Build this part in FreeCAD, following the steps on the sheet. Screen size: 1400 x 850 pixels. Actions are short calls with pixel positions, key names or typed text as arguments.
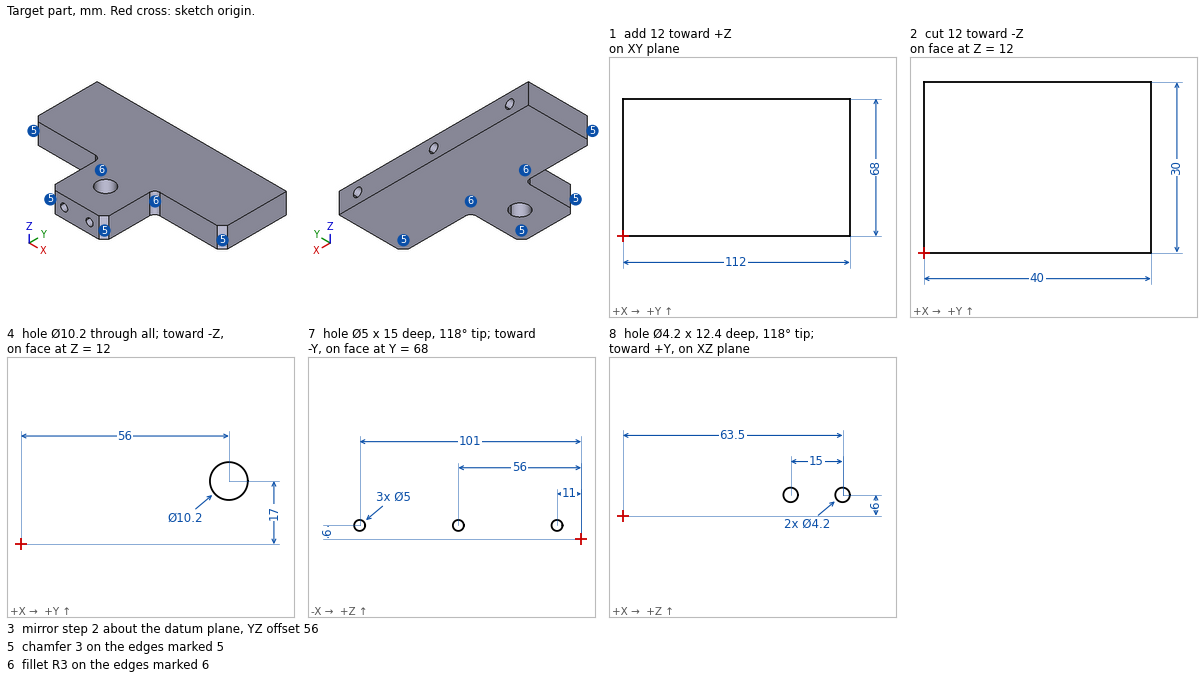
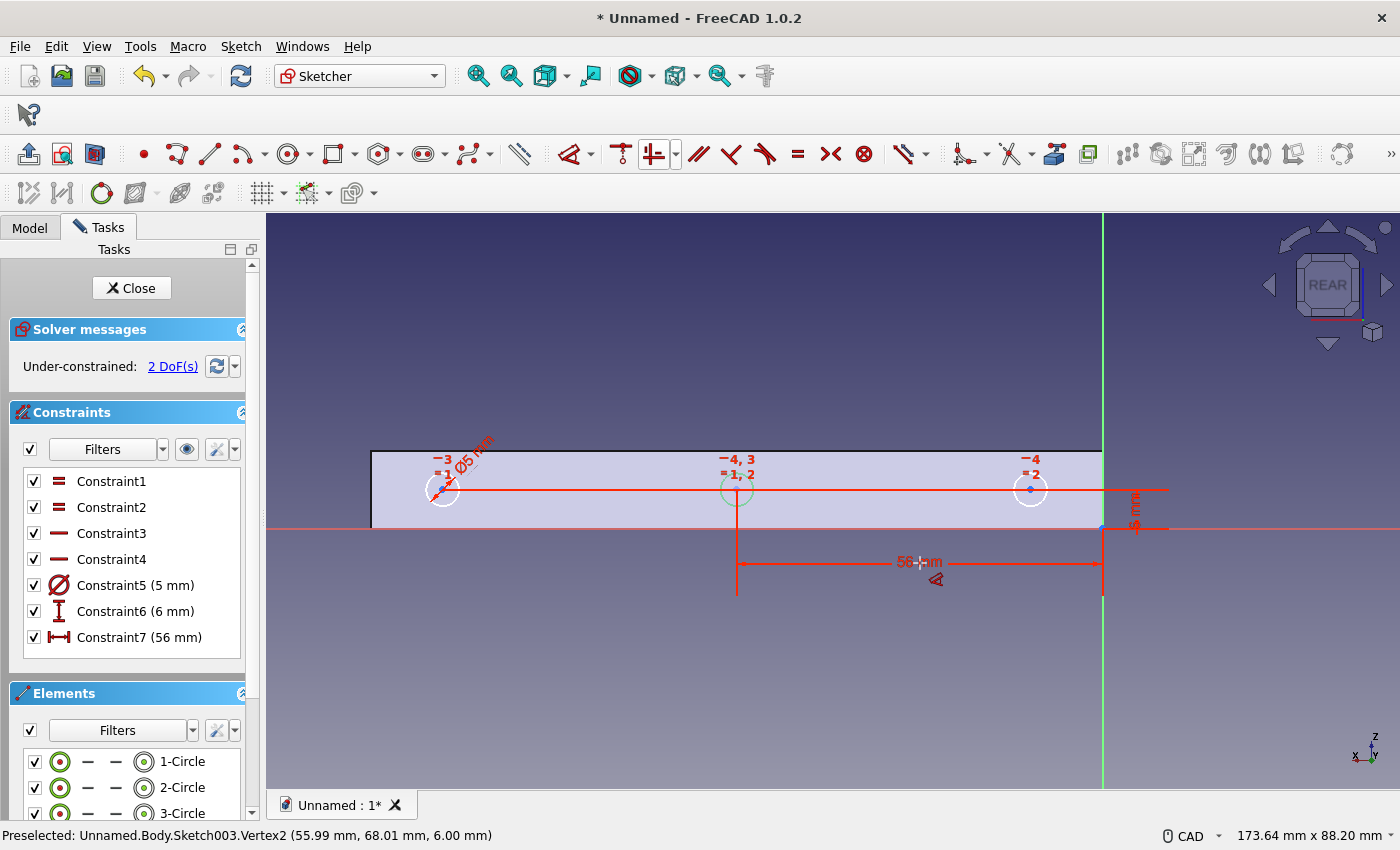
click(1031, 490)
click(1067, 563)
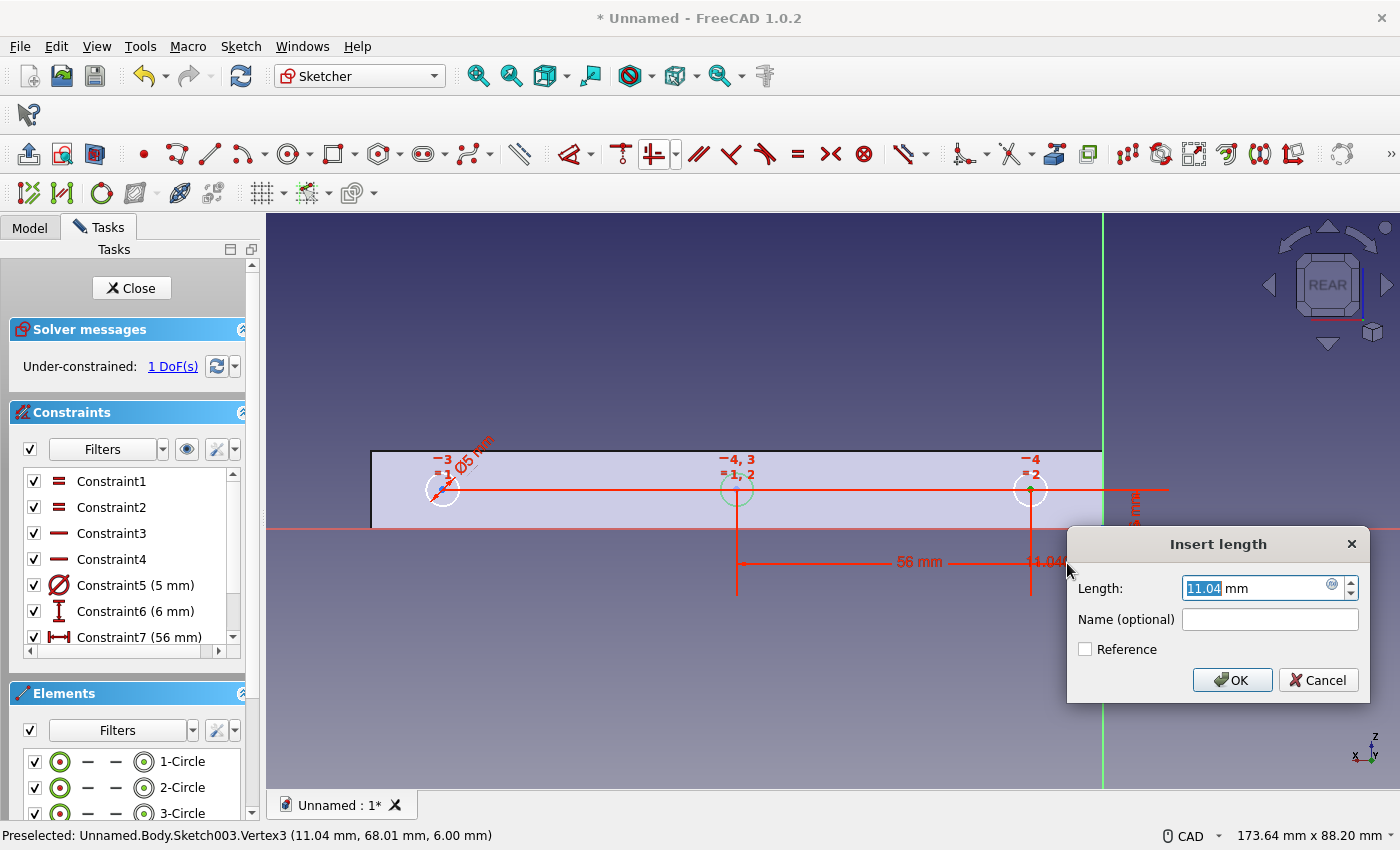
text(11)
key(Return)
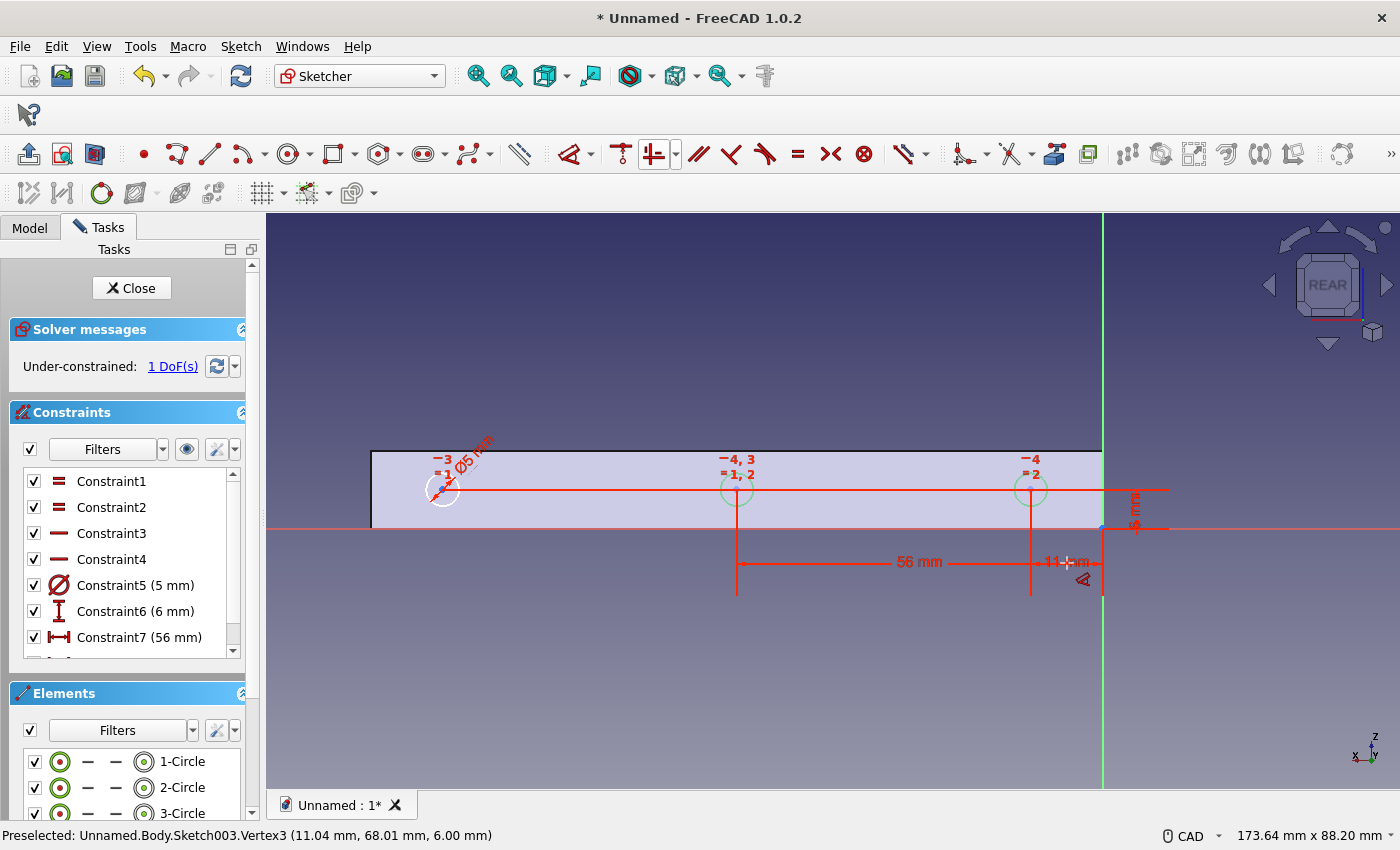
click(443, 490)
click(773, 563)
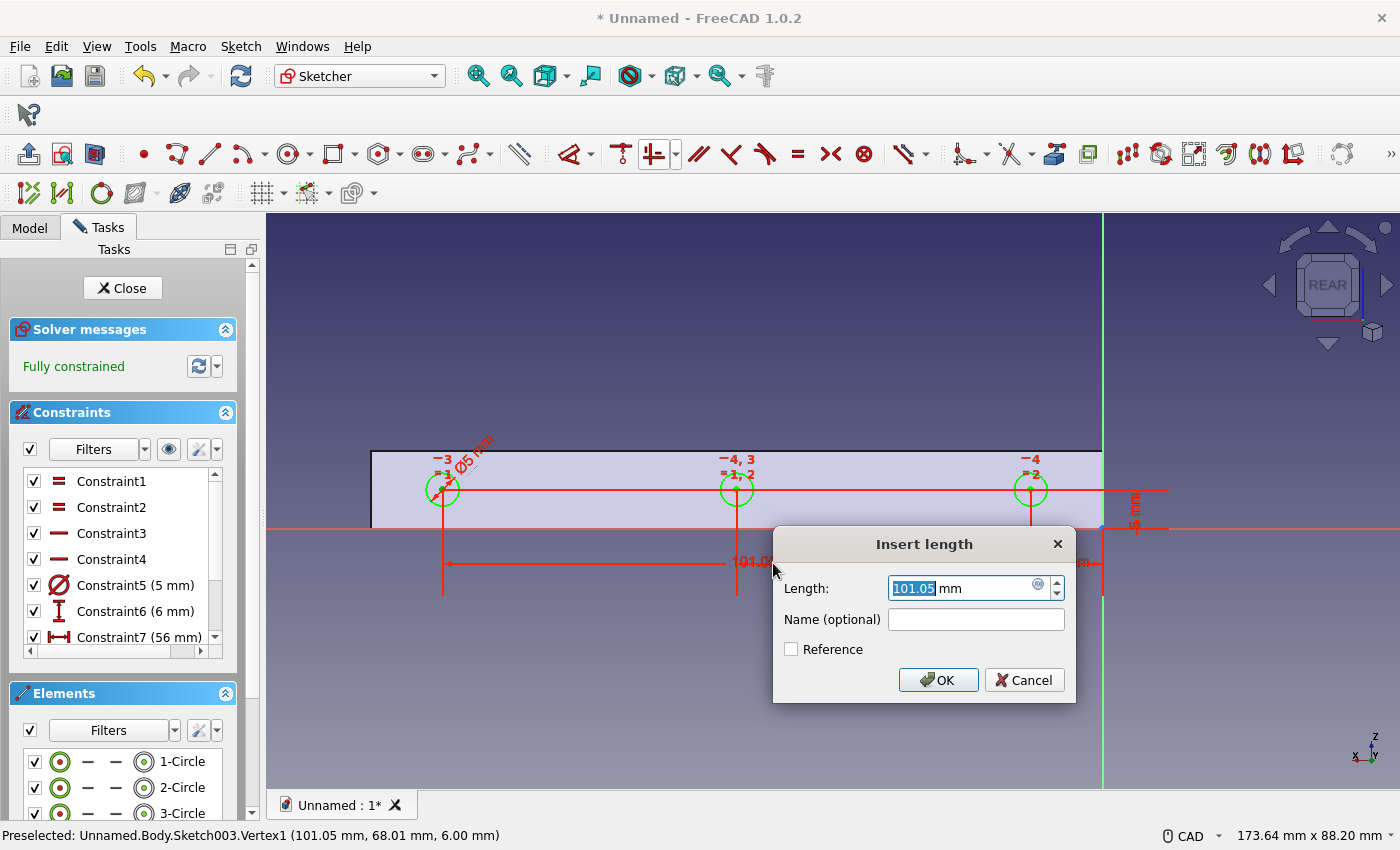
text(101)
key(Return)
key(Escape)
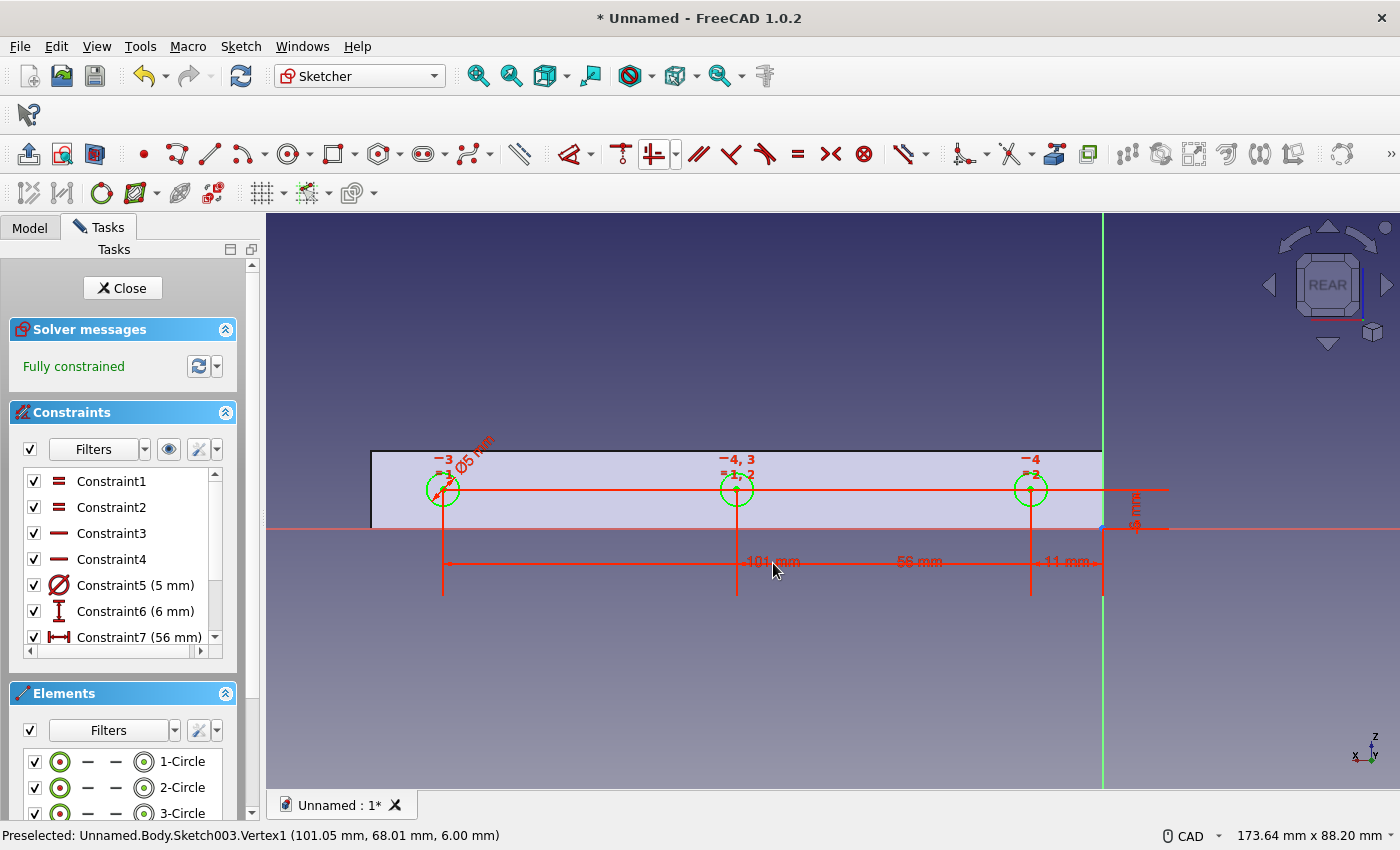
click(123, 288)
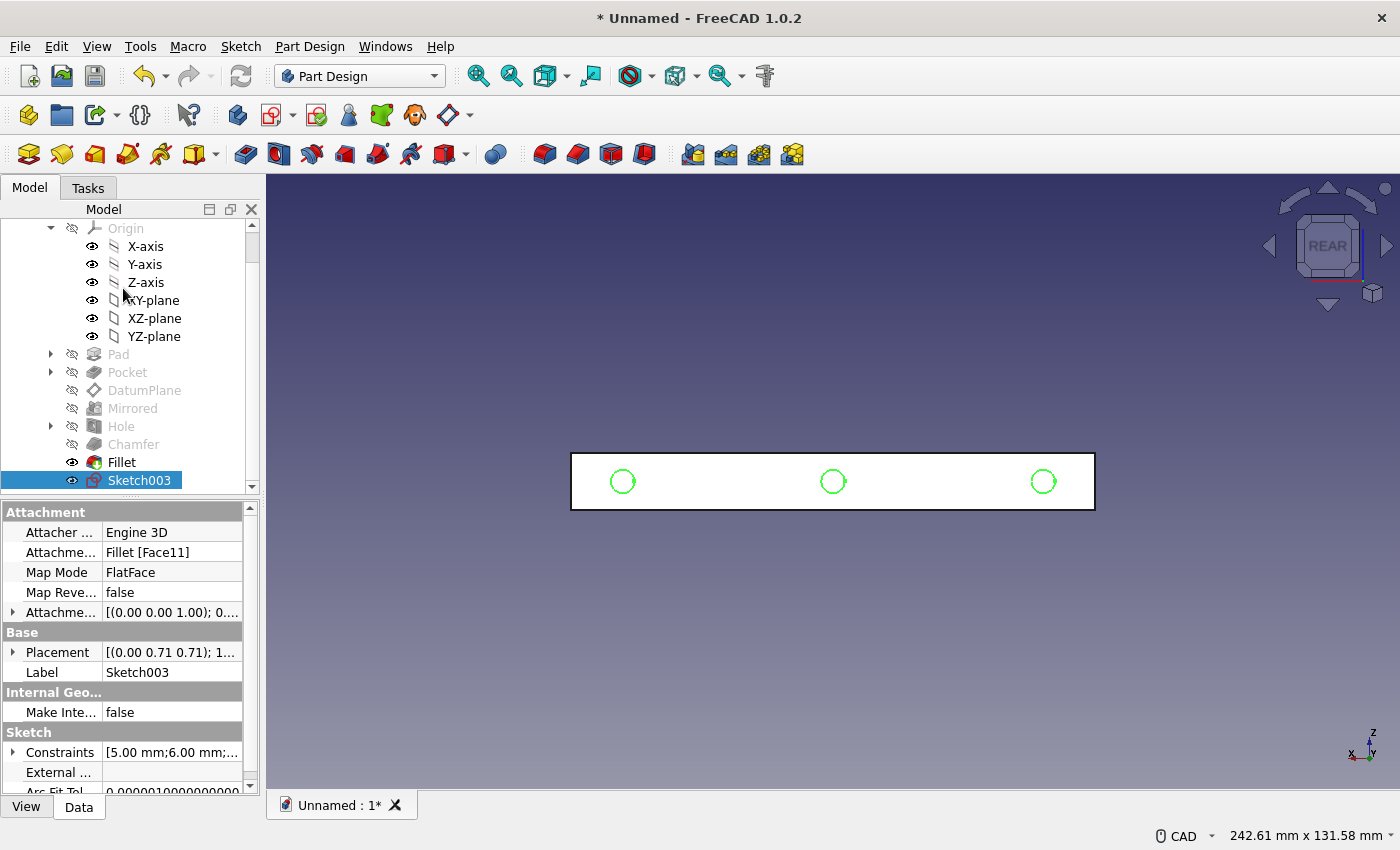
click(279, 154)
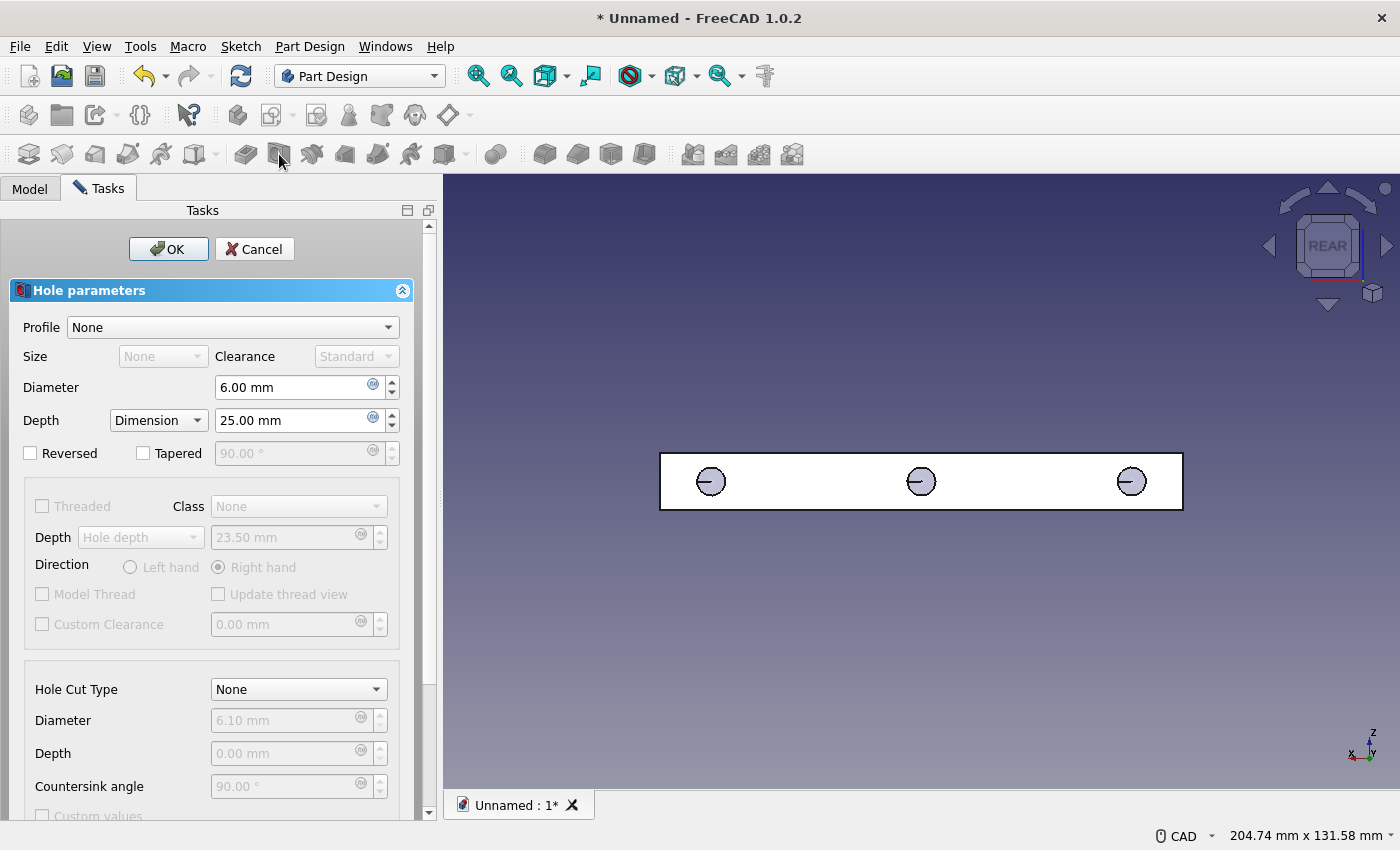
triple_click(300, 388)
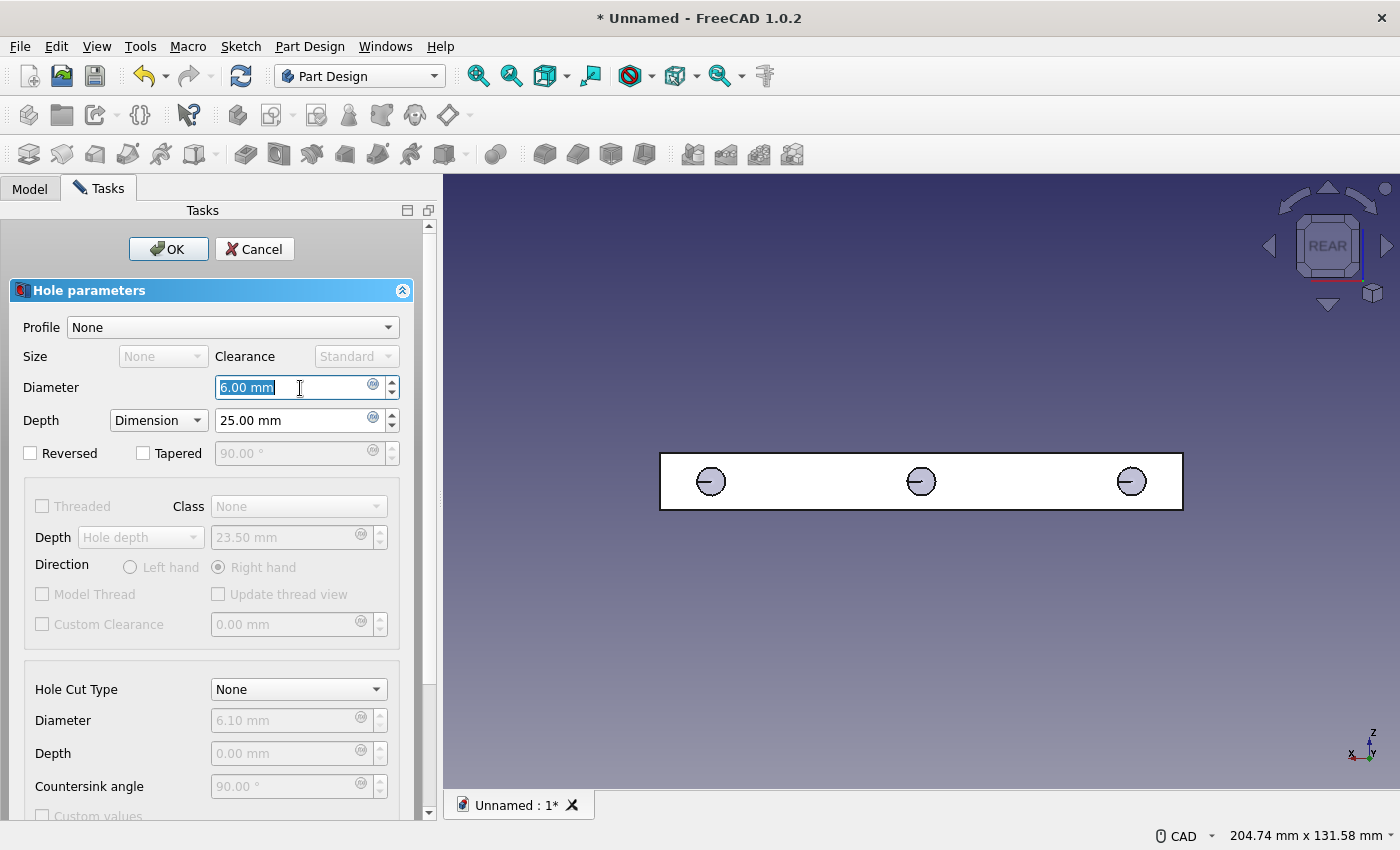
text(5)
key(Tab)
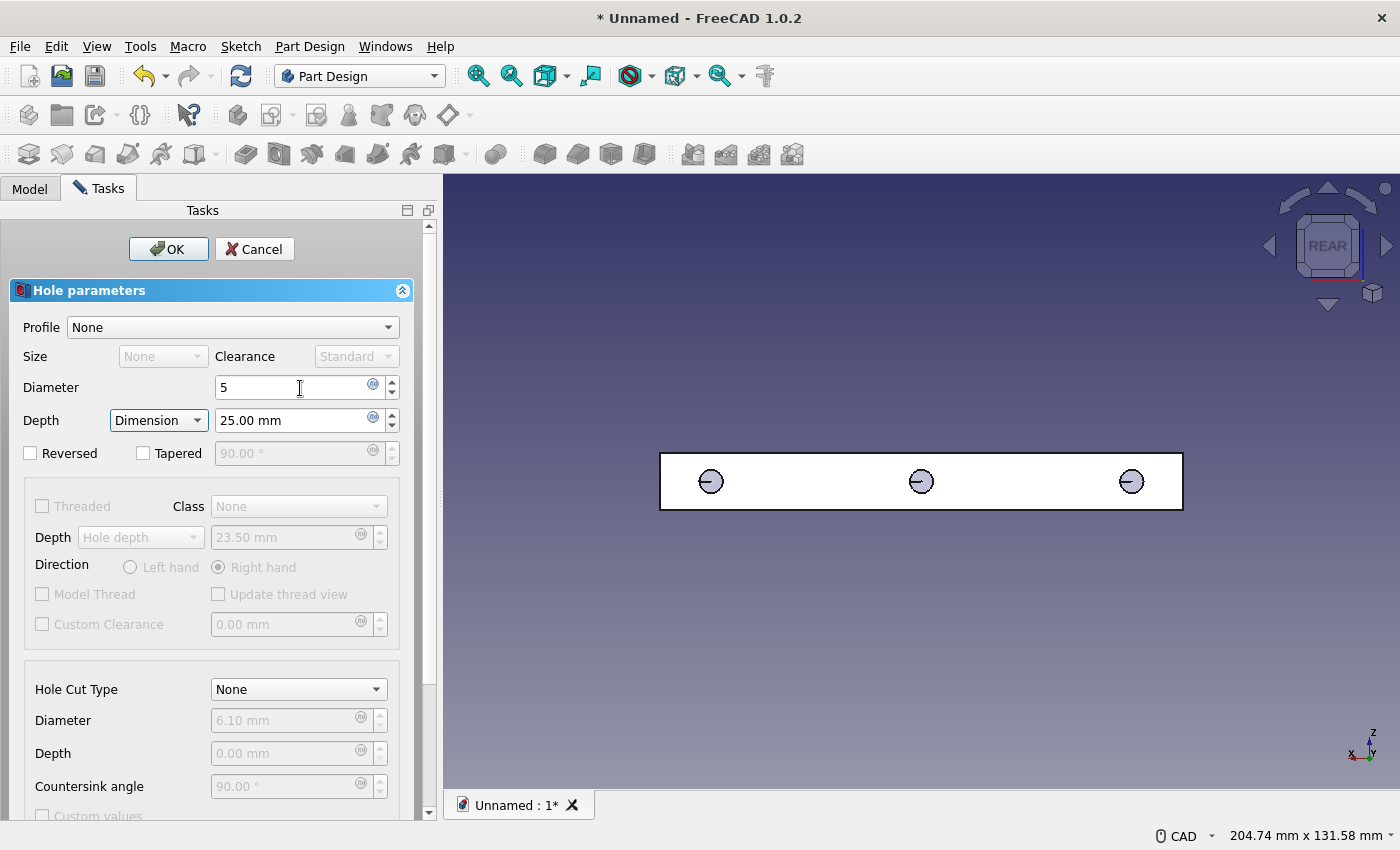
triple_click(300, 420)